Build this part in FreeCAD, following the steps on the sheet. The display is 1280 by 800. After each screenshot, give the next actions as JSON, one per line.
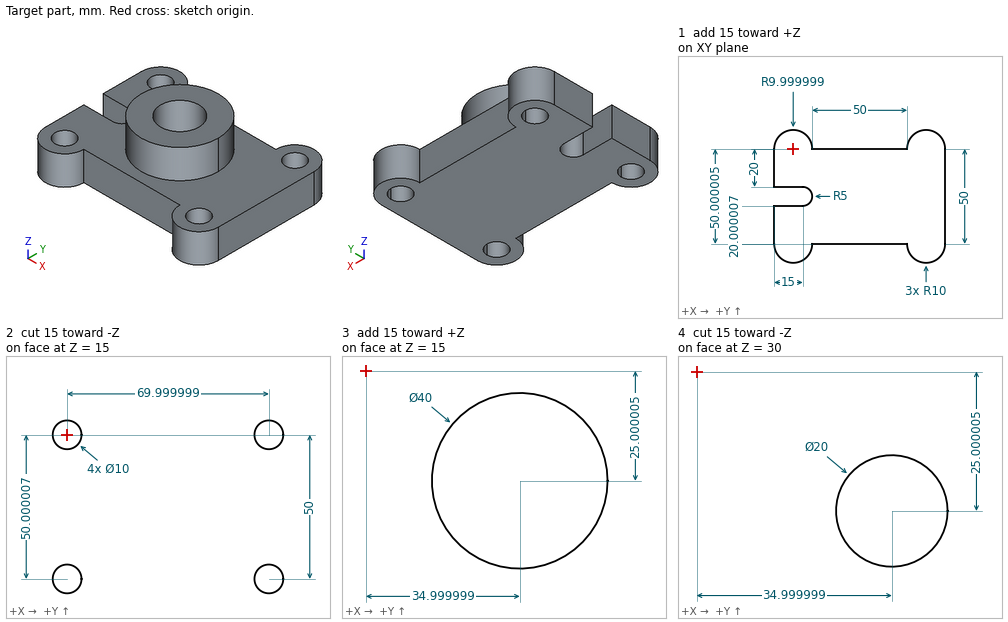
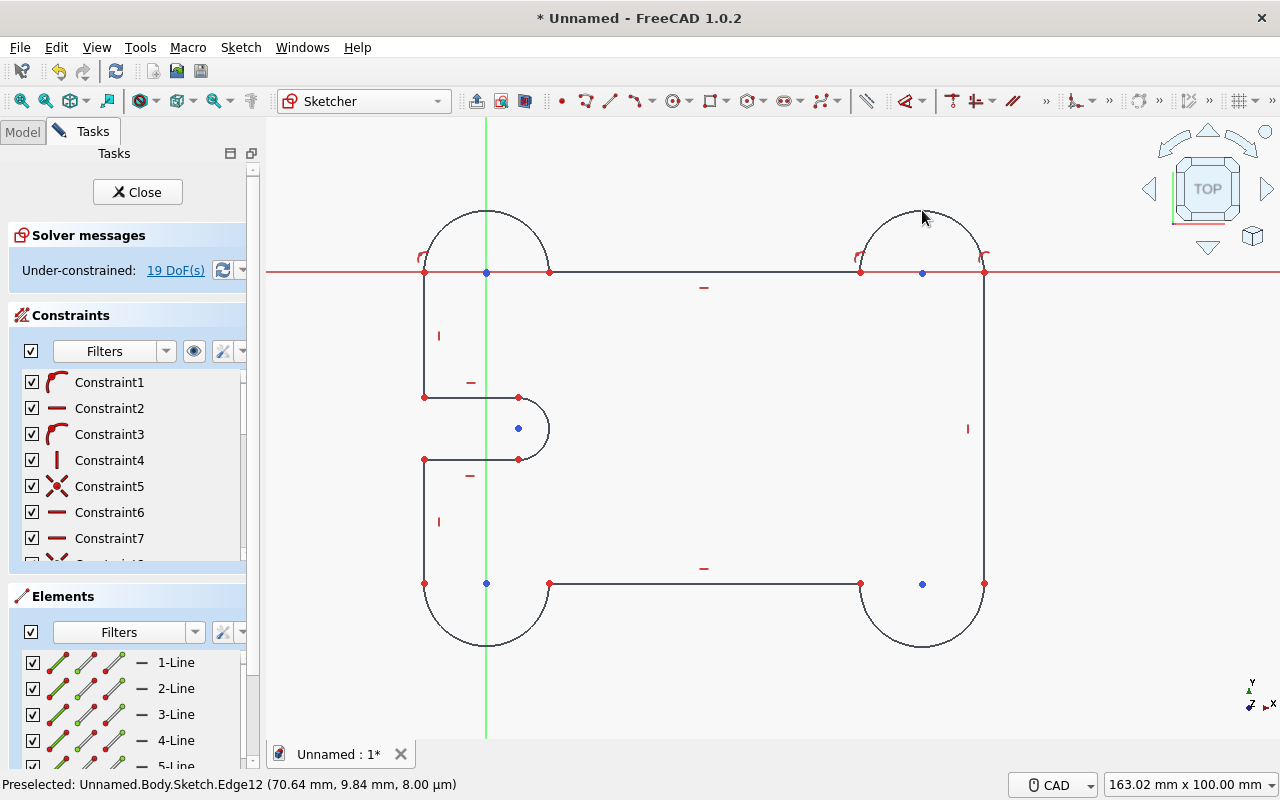
{"action": "left_click", "coordinate": [424, 310]}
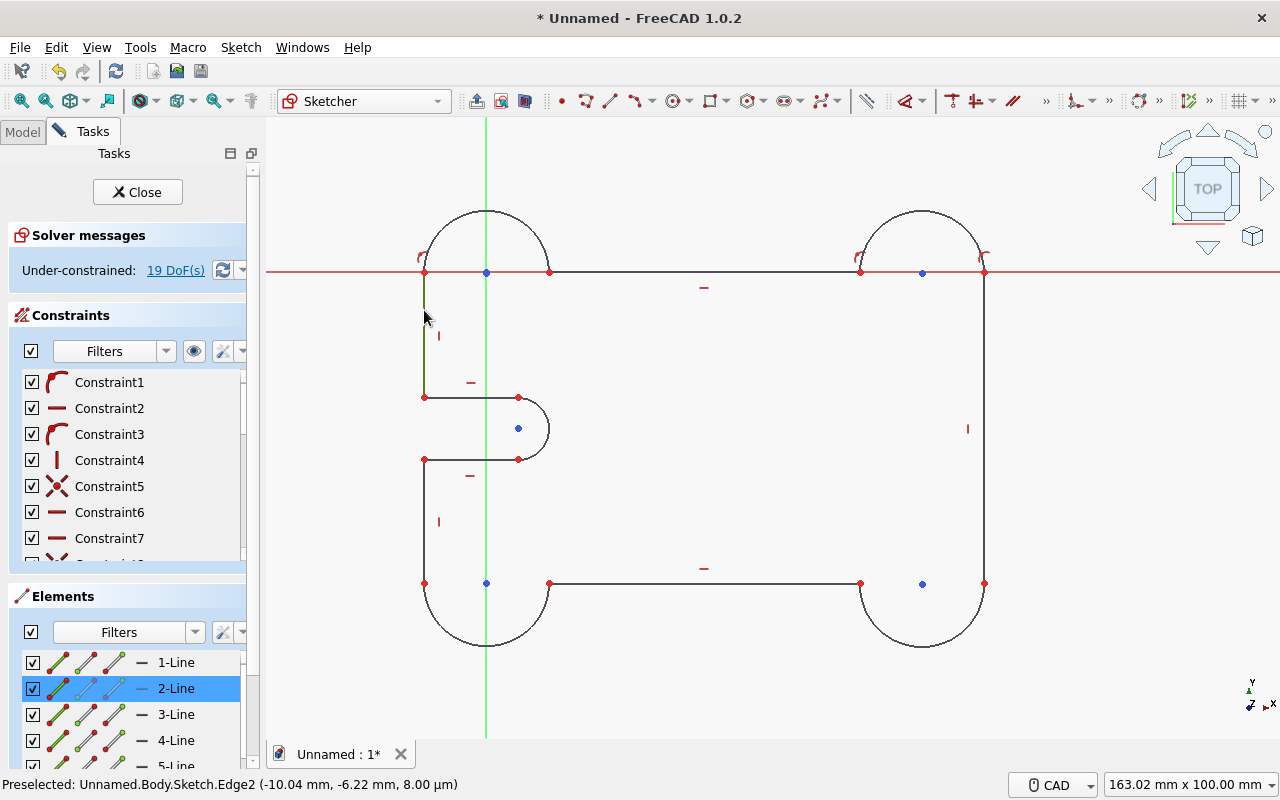
{"action": "left_click", "coordinate": [523, 223]}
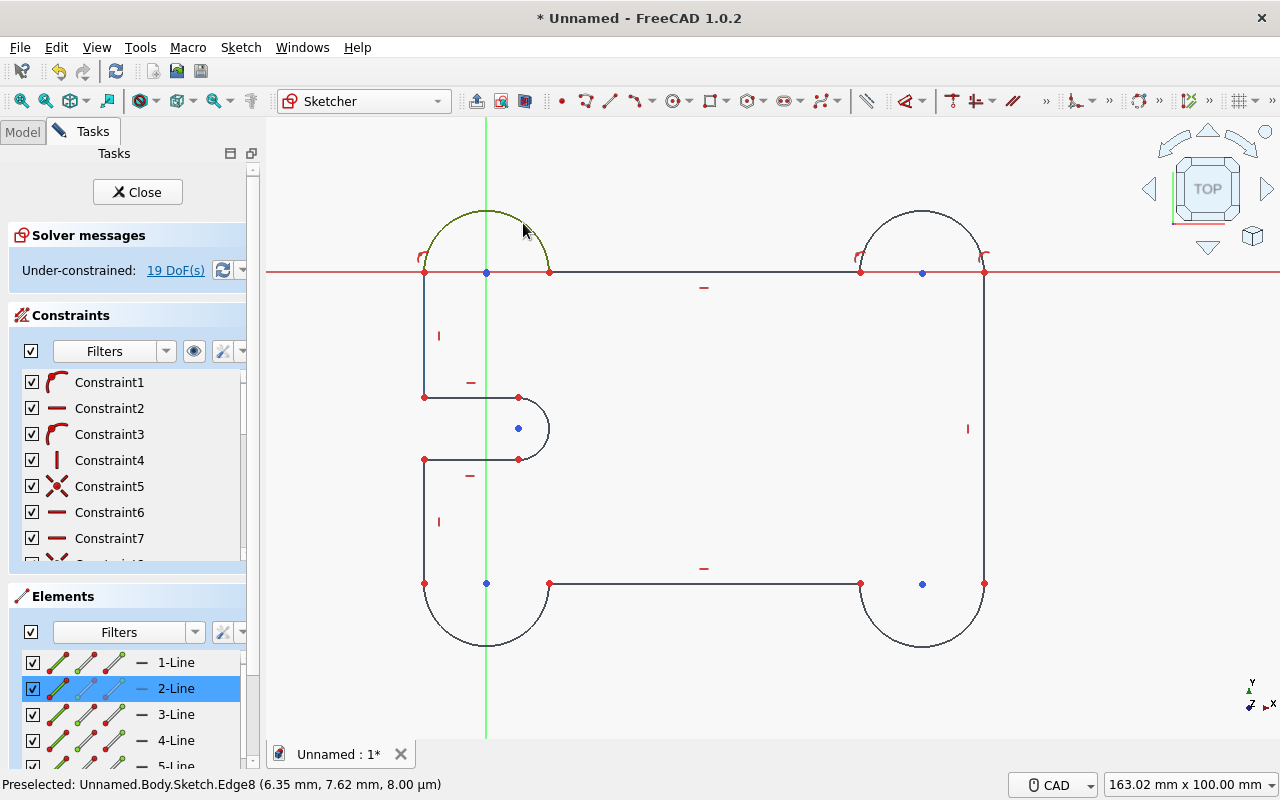
{"action": "key", "text": "t"}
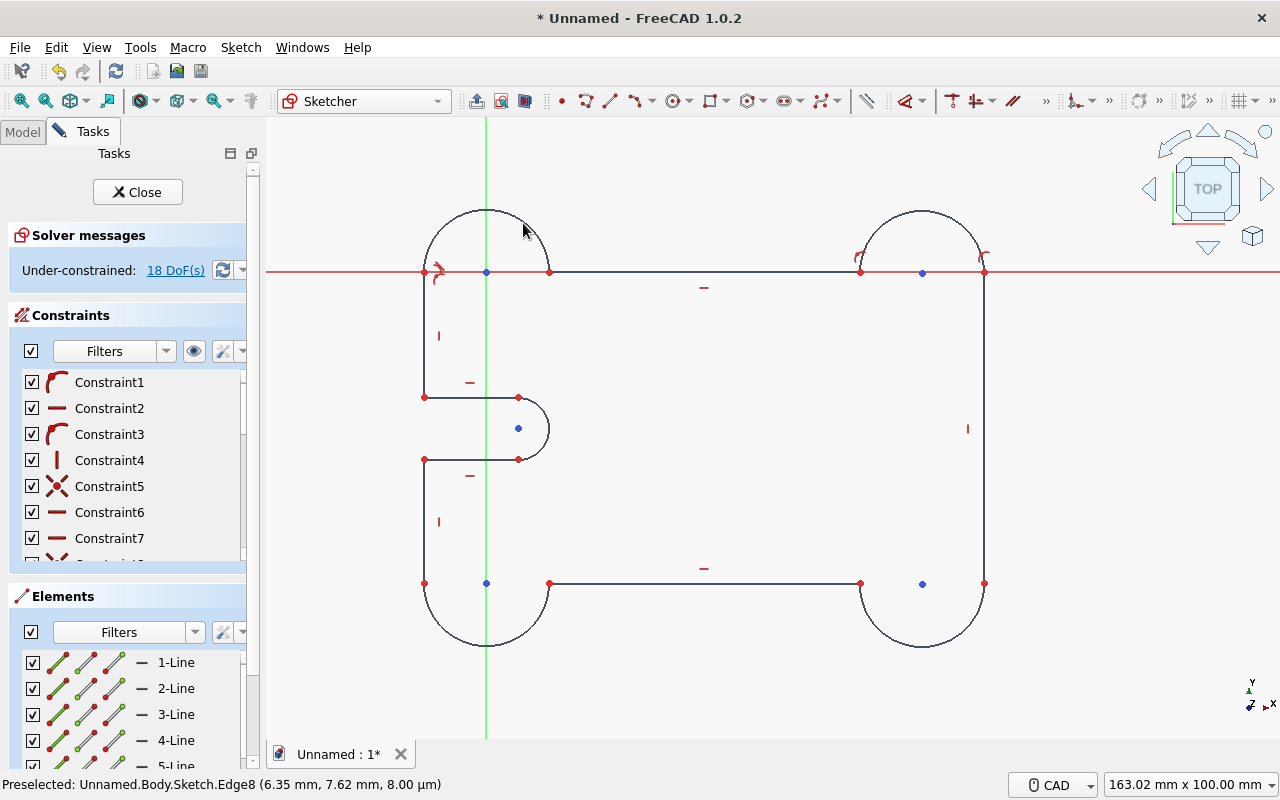
{"action": "left_click", "coordinate": [452, 398]}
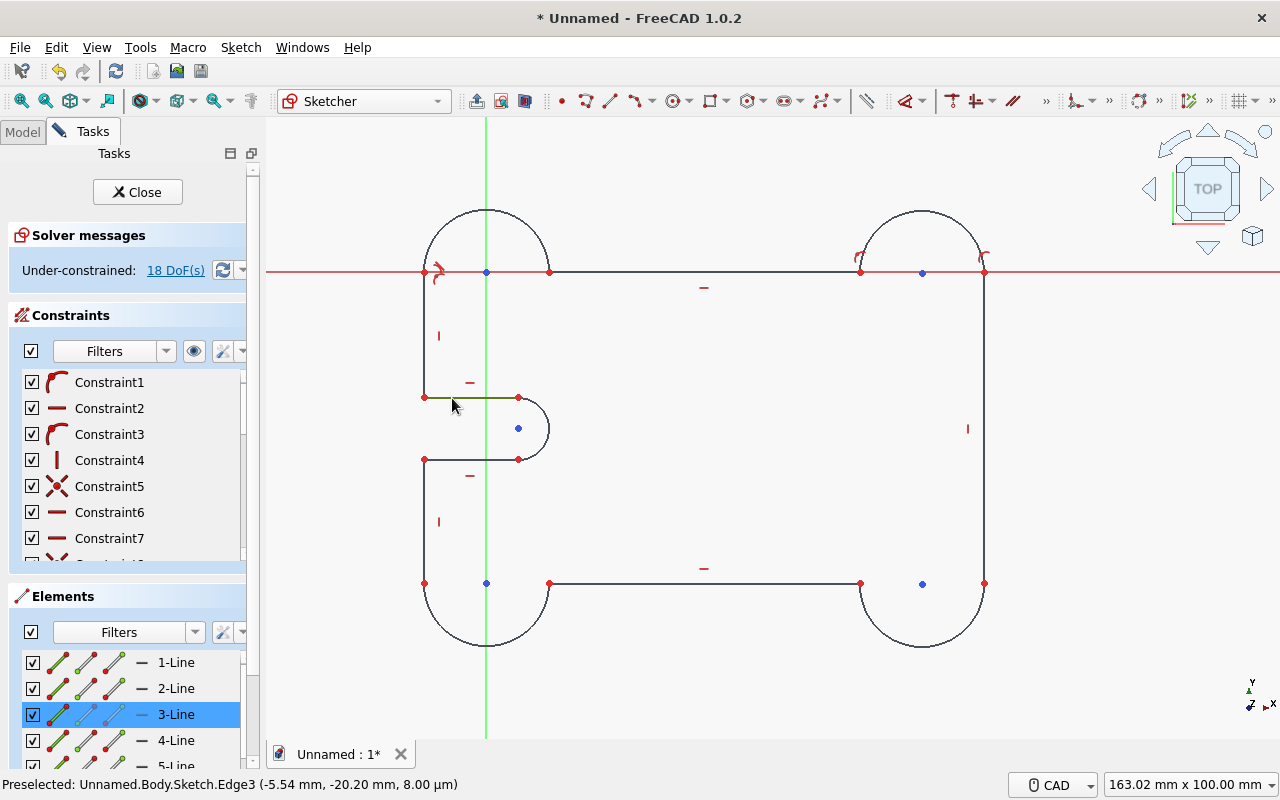
{"action": "left_click", "coordinate": [543, 447]}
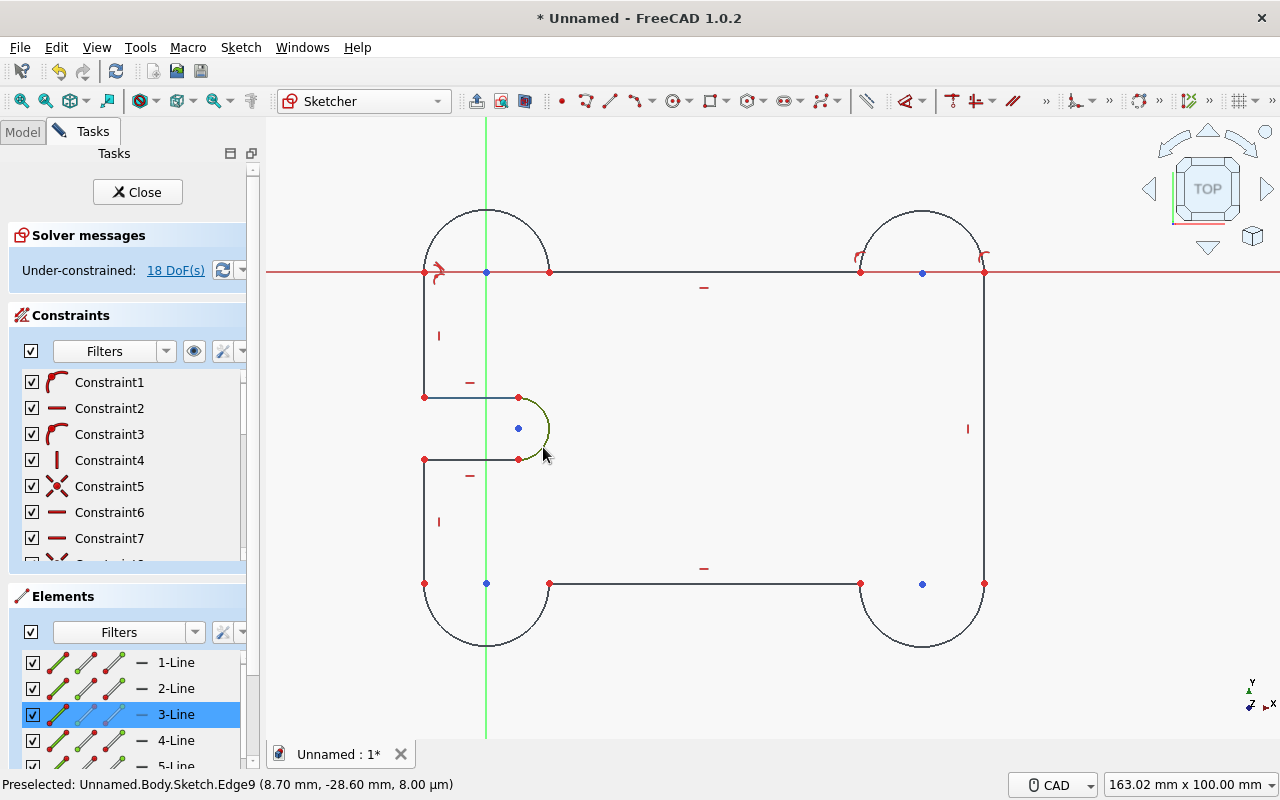
{"action": "key", "text": "t"}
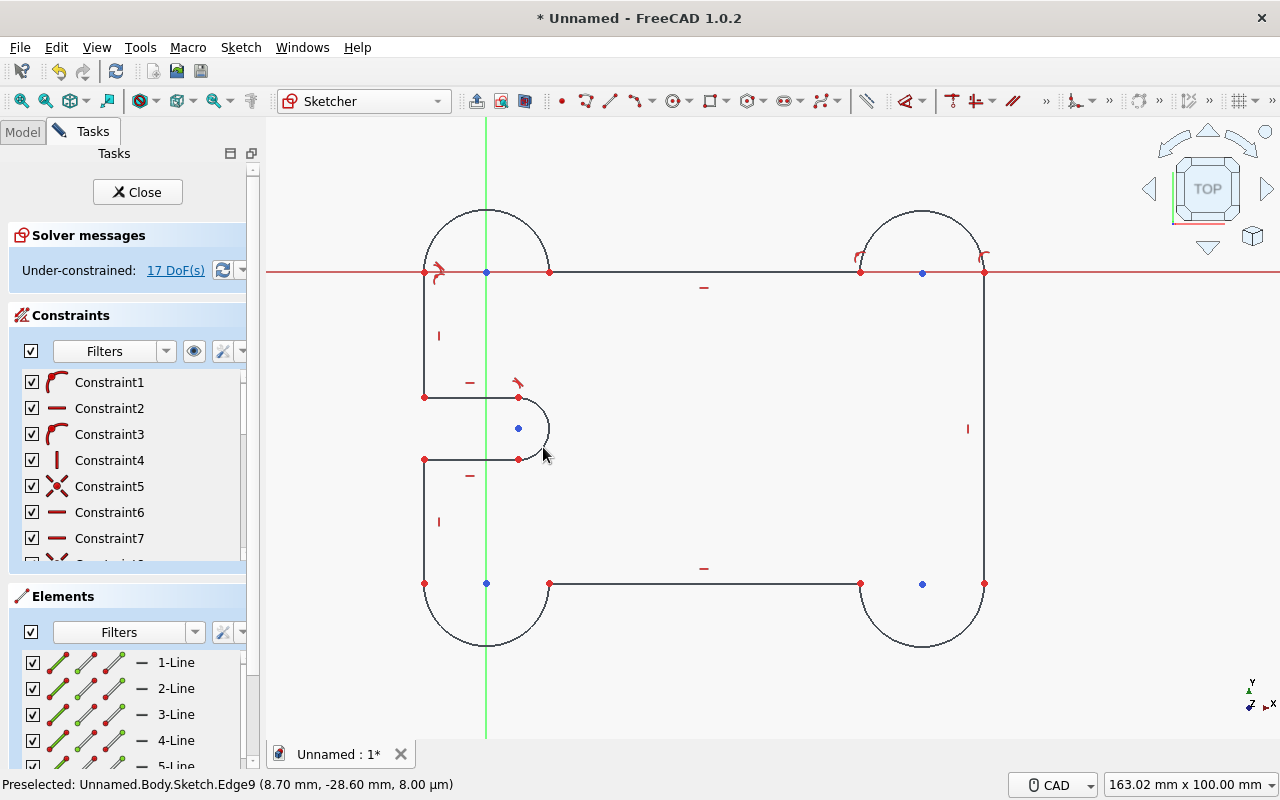
{"action": "left_click", "coordinate": [490, 460]}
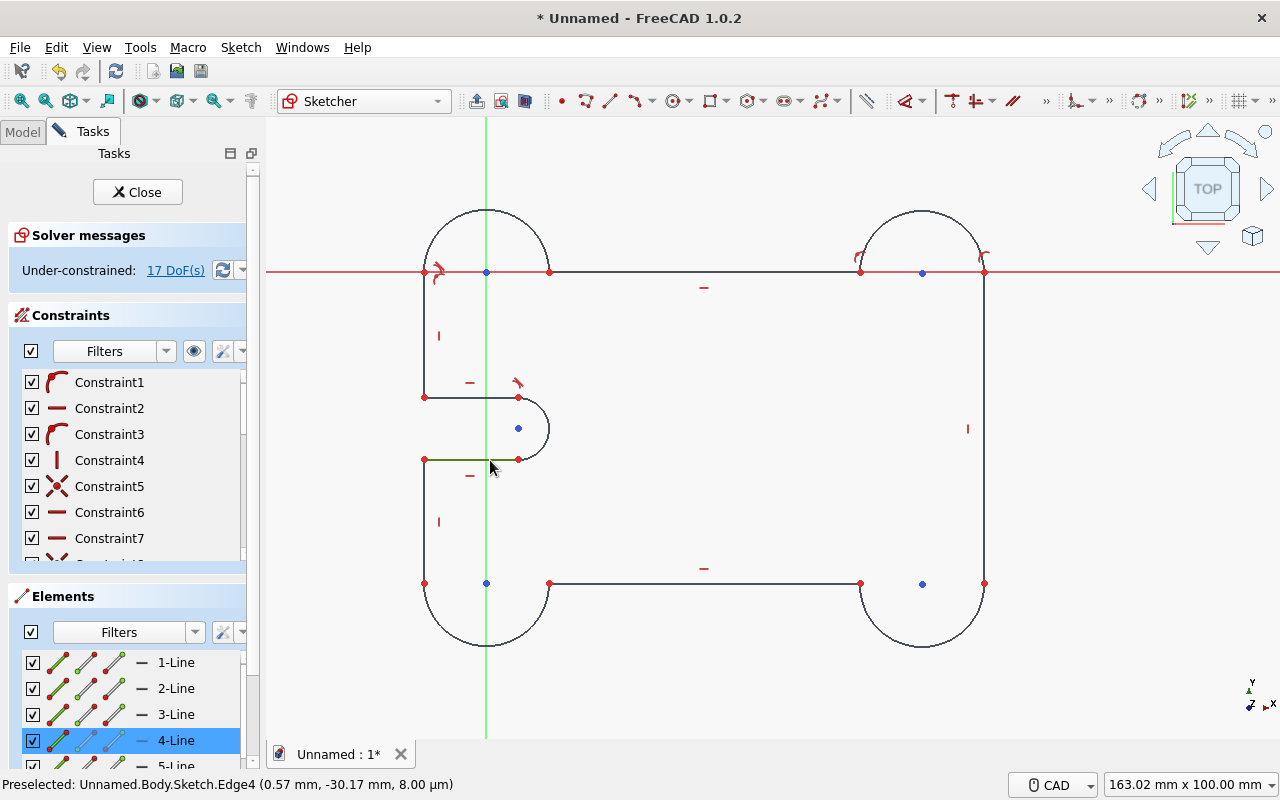
{"action": "left_click", "coordinate": [543, 447]}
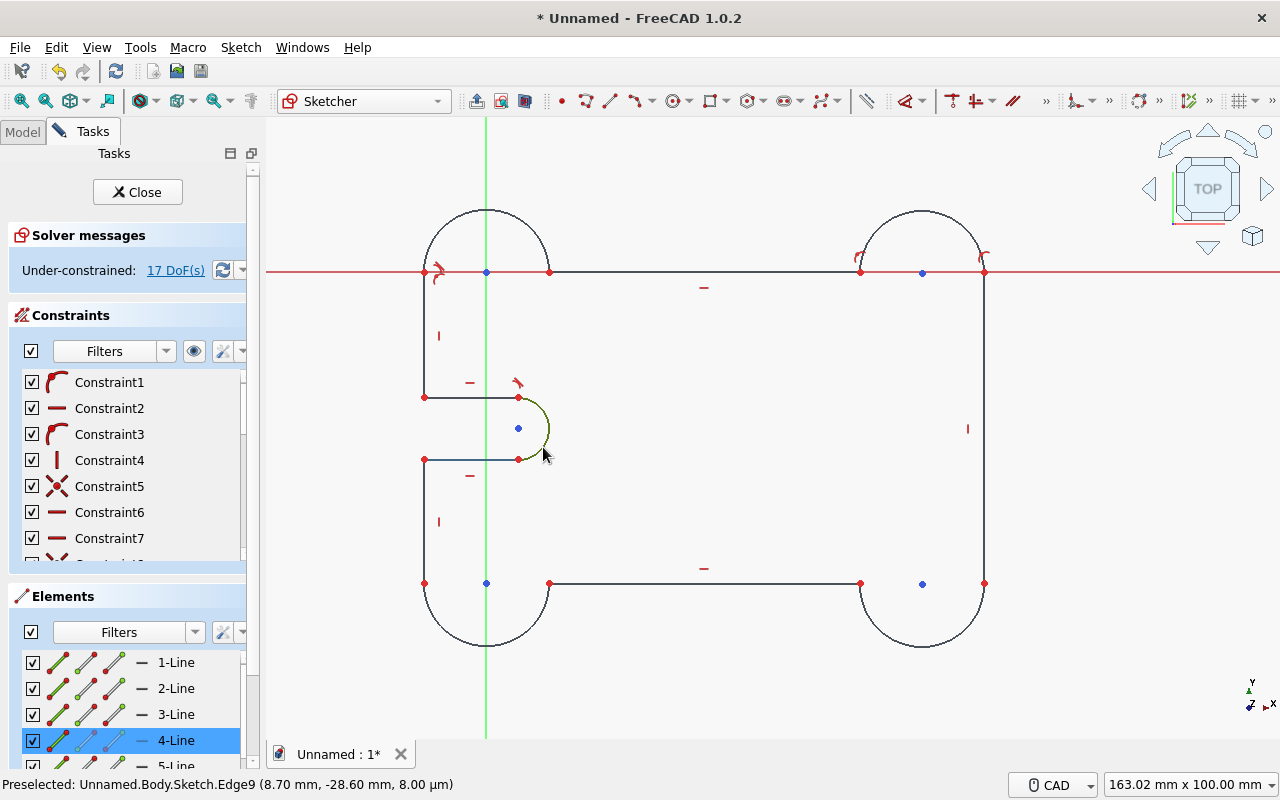
{"action": "key", "text": "t"}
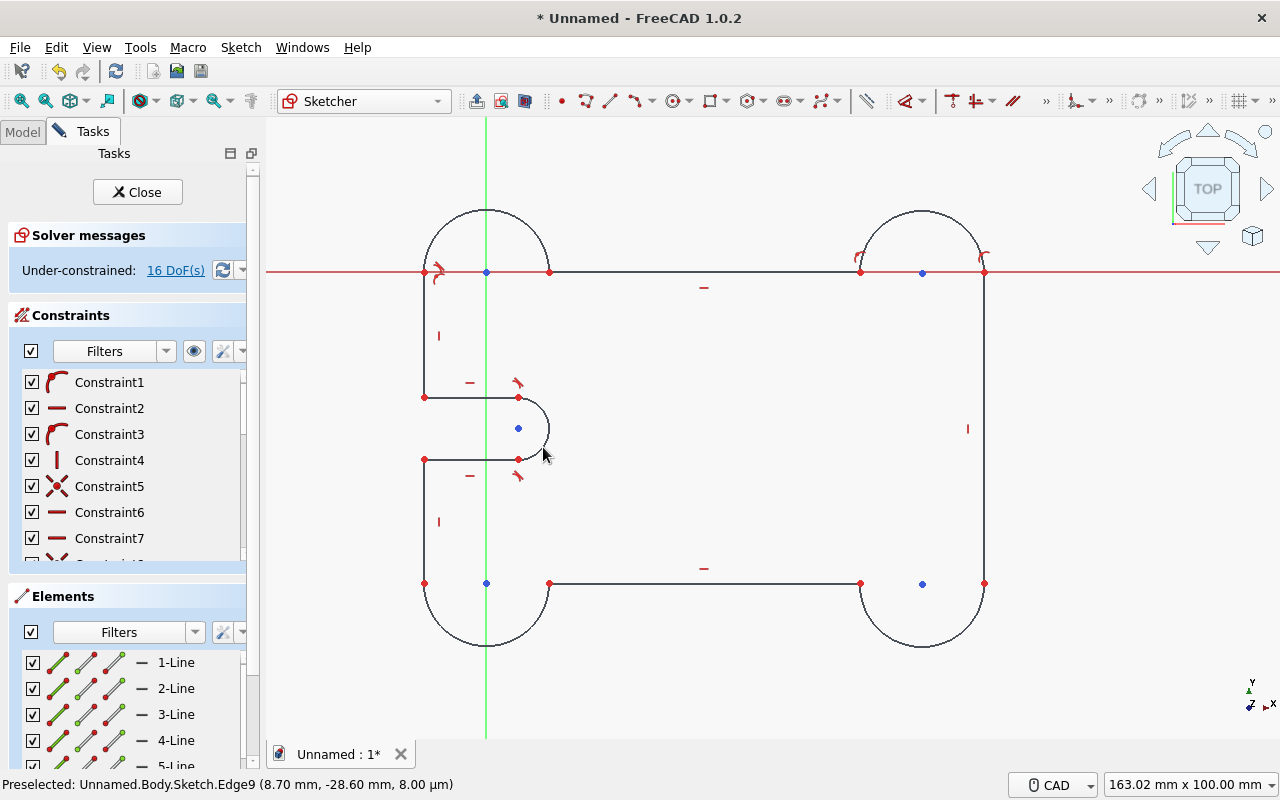
{"action": "left_click", "coordinate": [424, 497]}